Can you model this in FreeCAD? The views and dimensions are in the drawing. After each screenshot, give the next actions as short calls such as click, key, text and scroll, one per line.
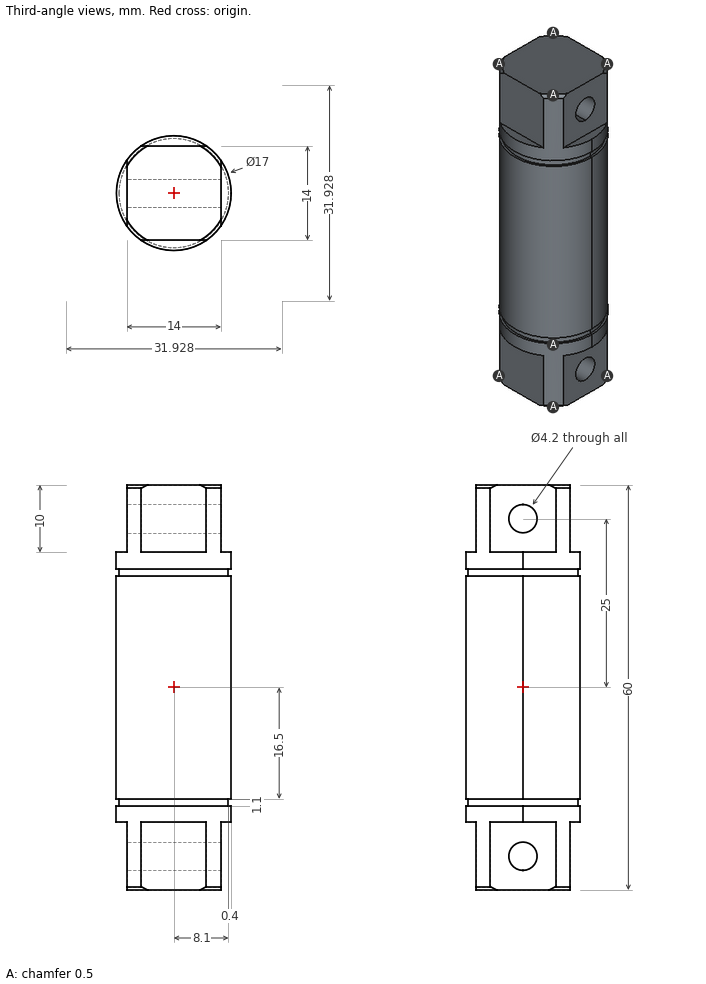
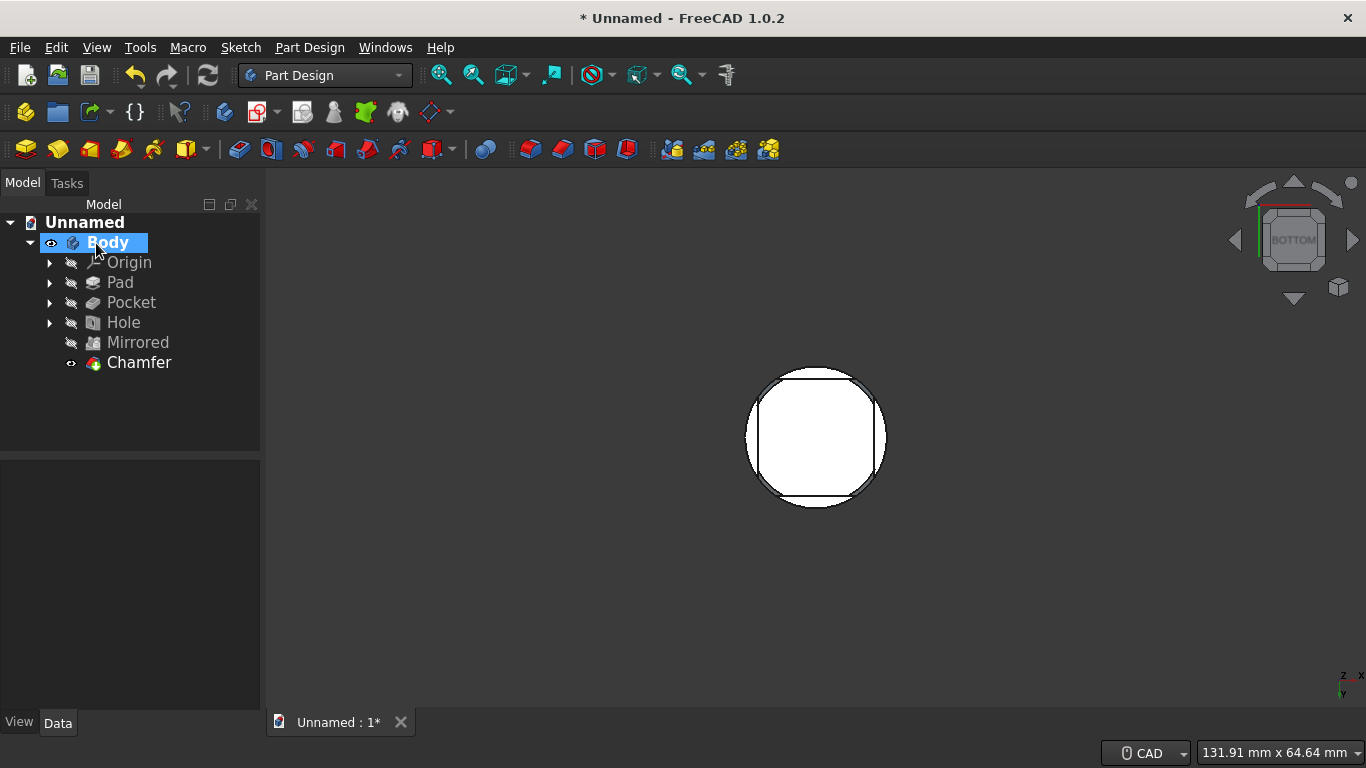
click(442, 76)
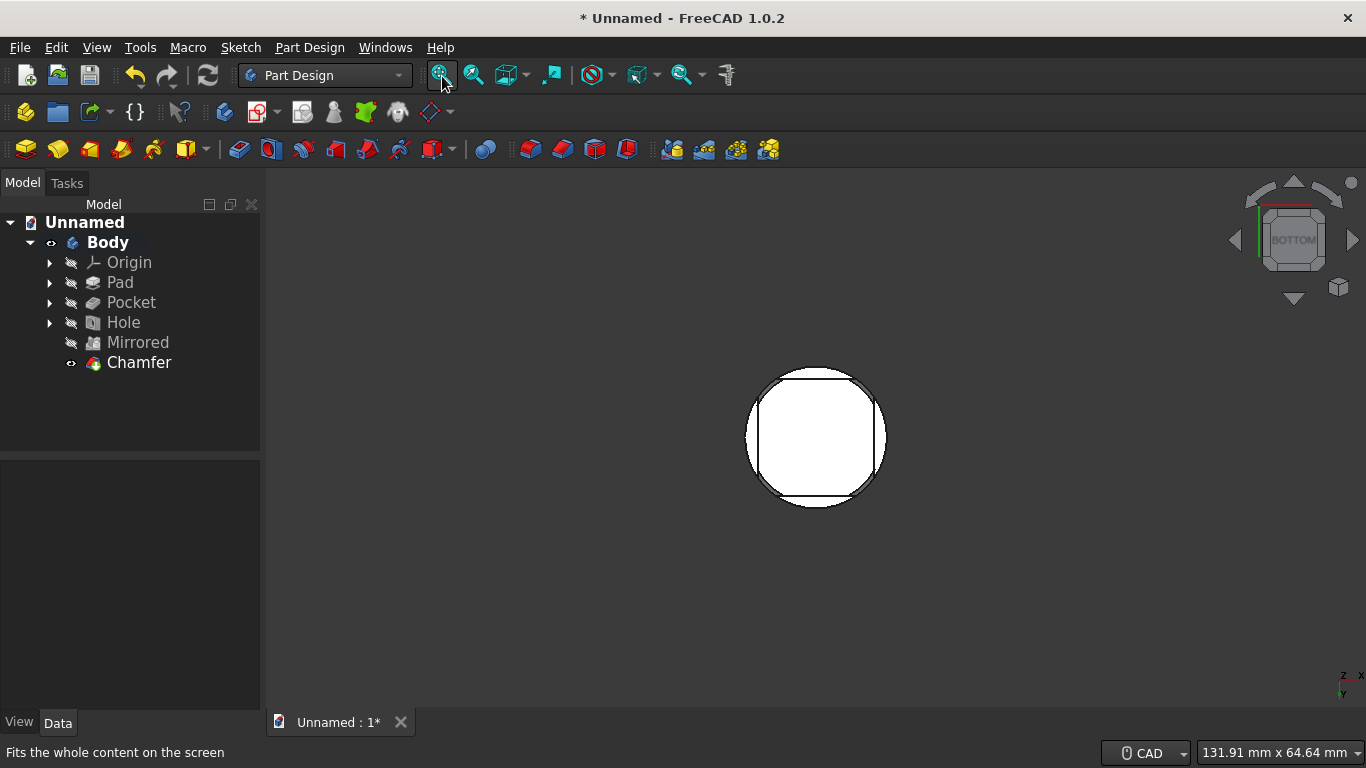
click(258, 112)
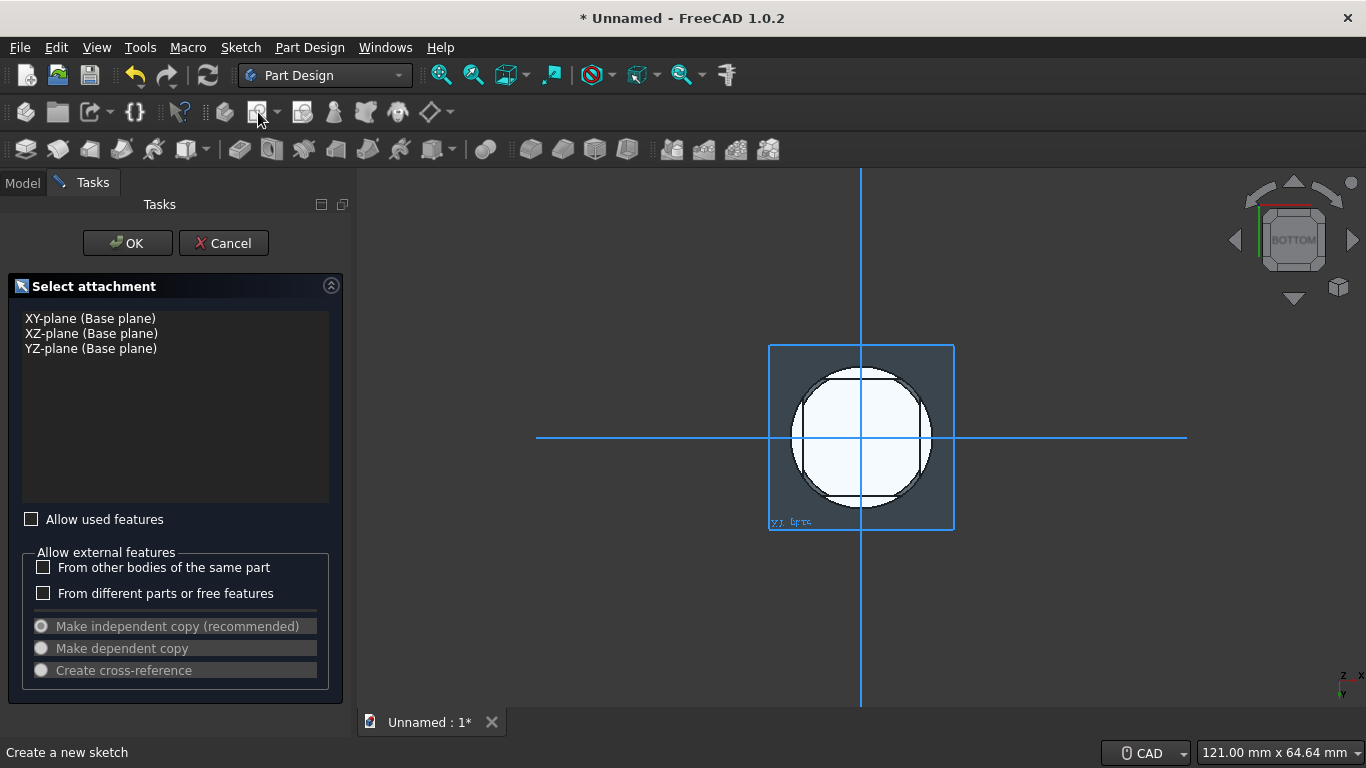
click(82, 334)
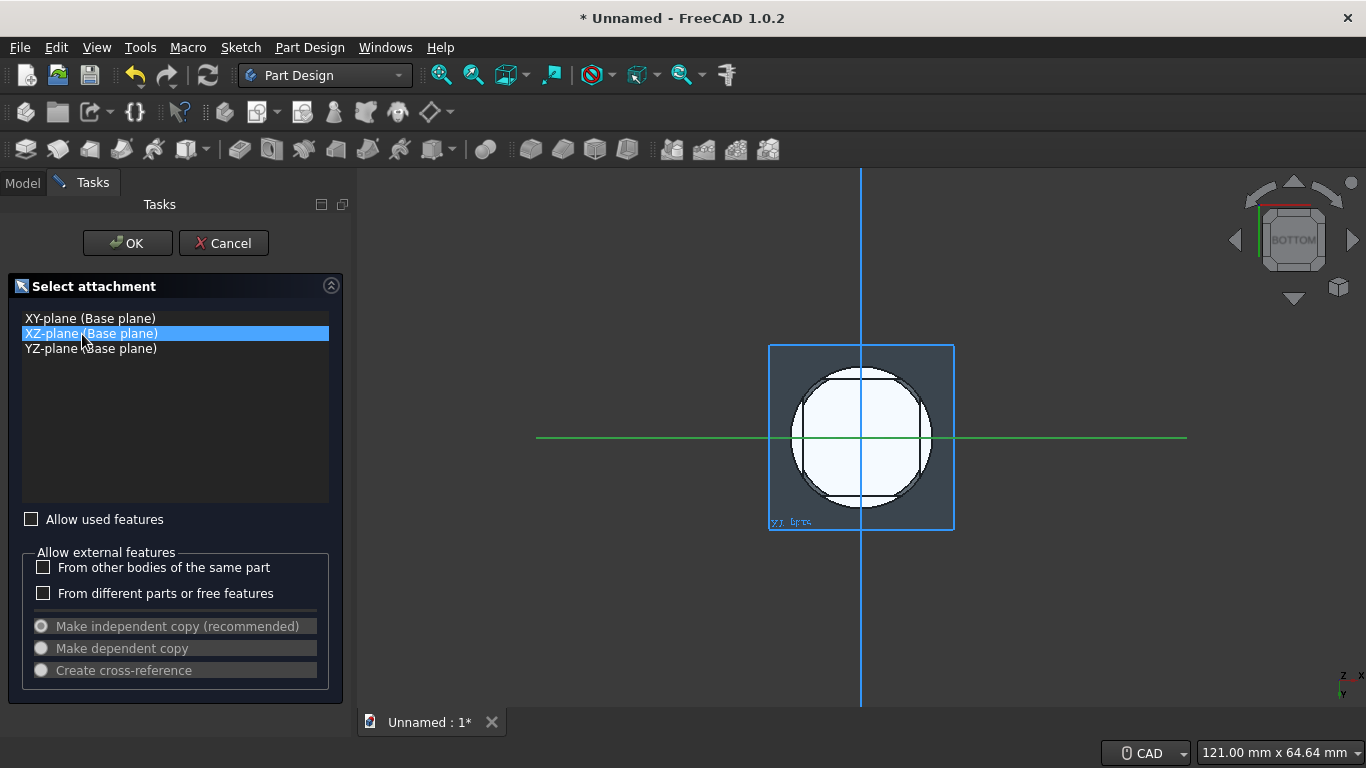
click(128, 243)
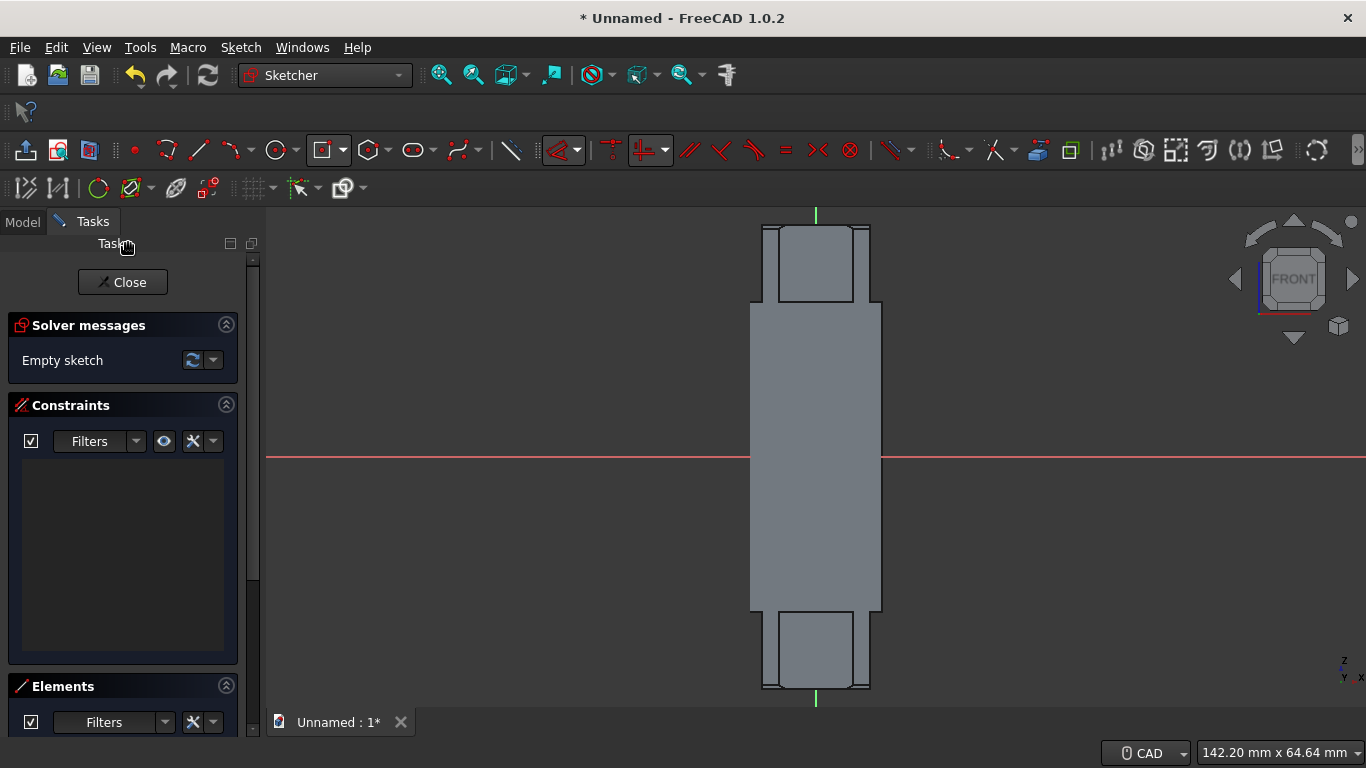
key(q)
key(s)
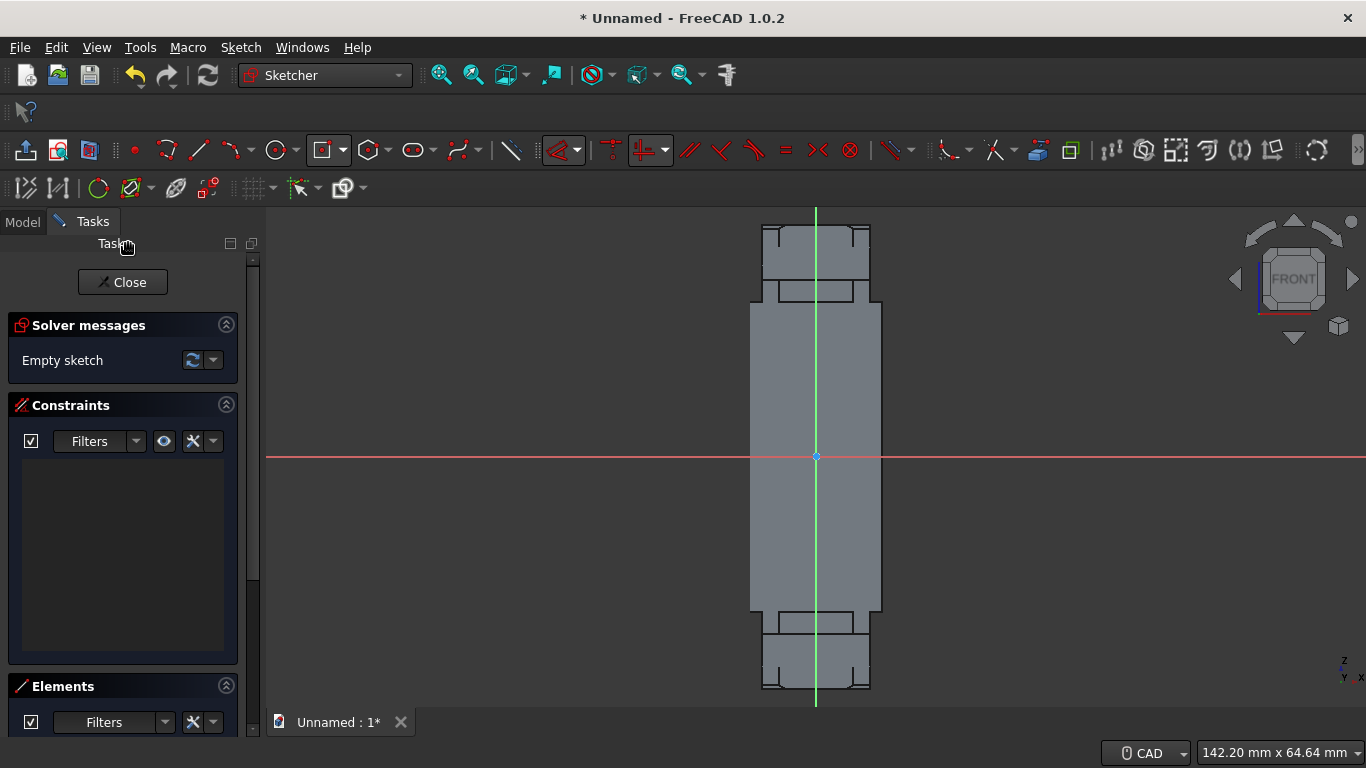
scroll(887, 596, up, 15)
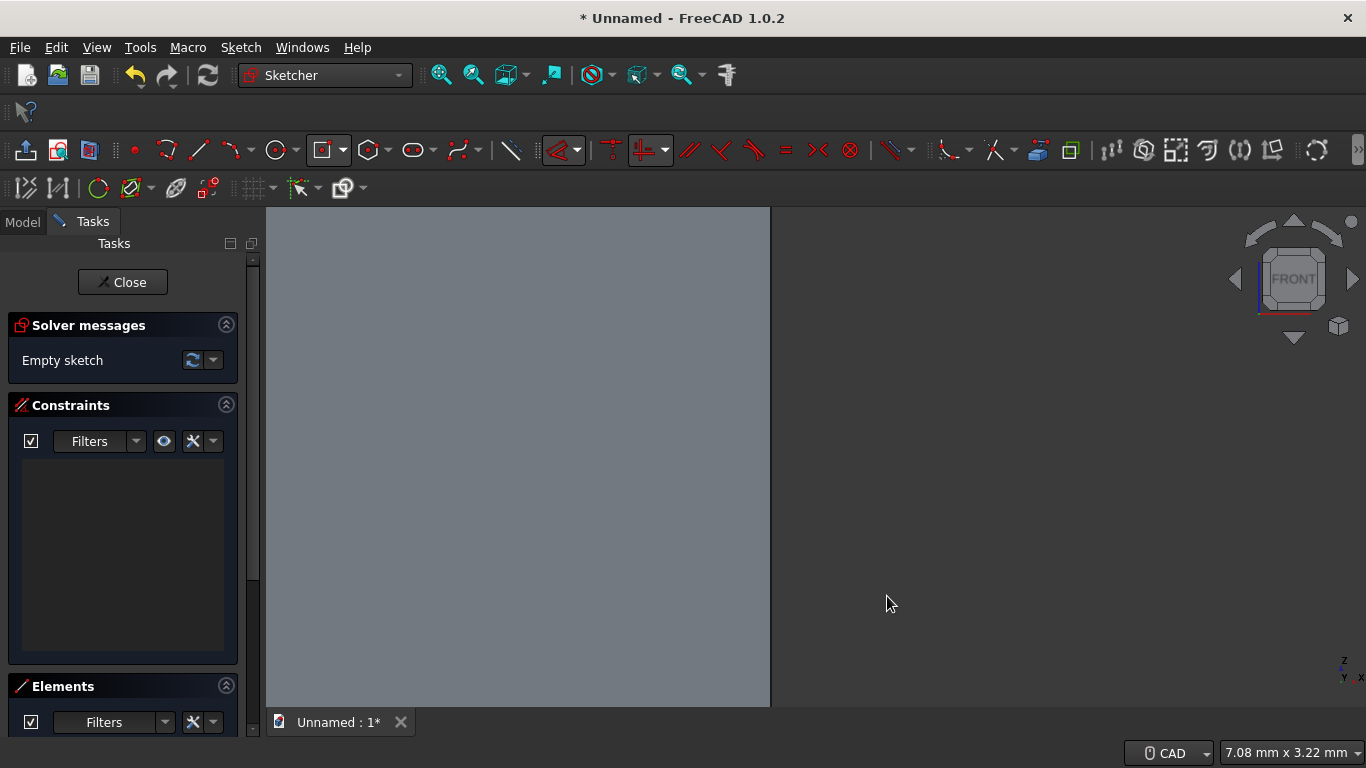
scroll(730, 416, up, 3)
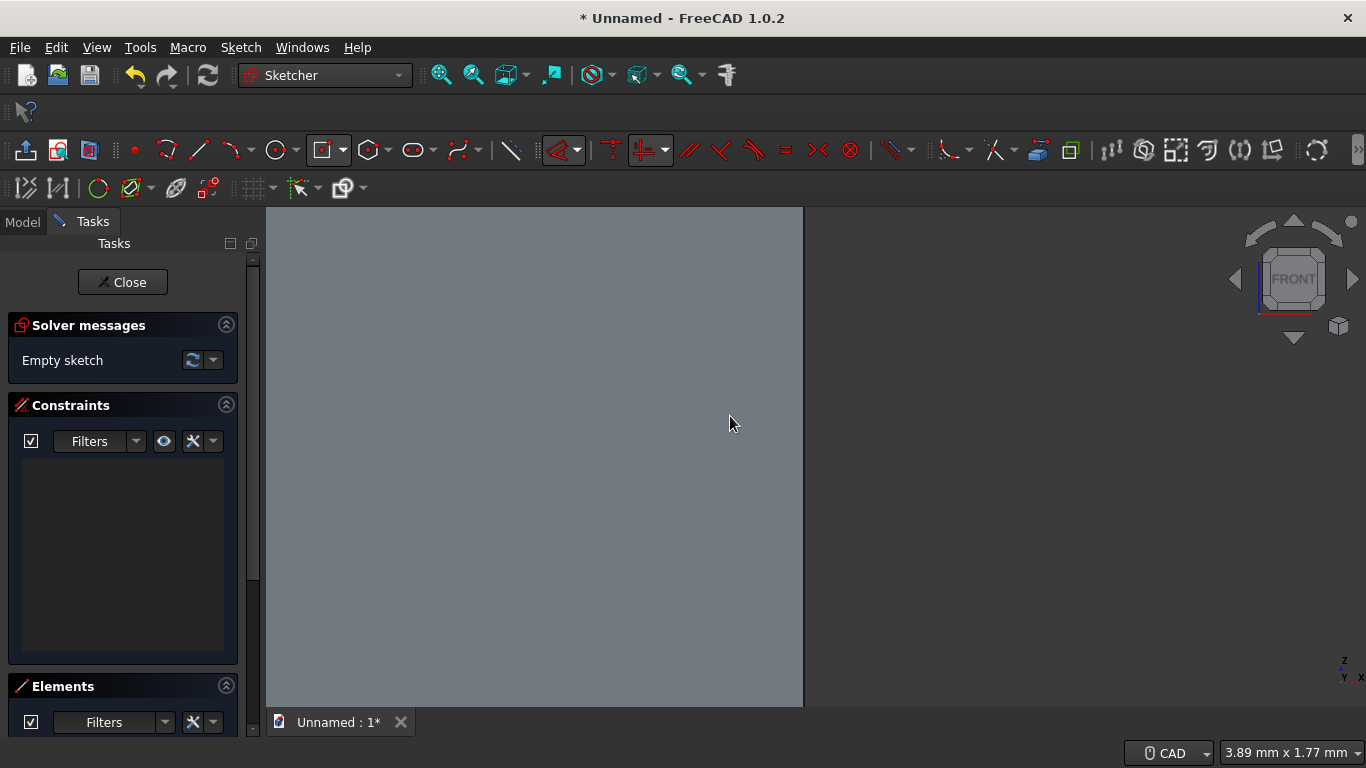
key(g)
key(r)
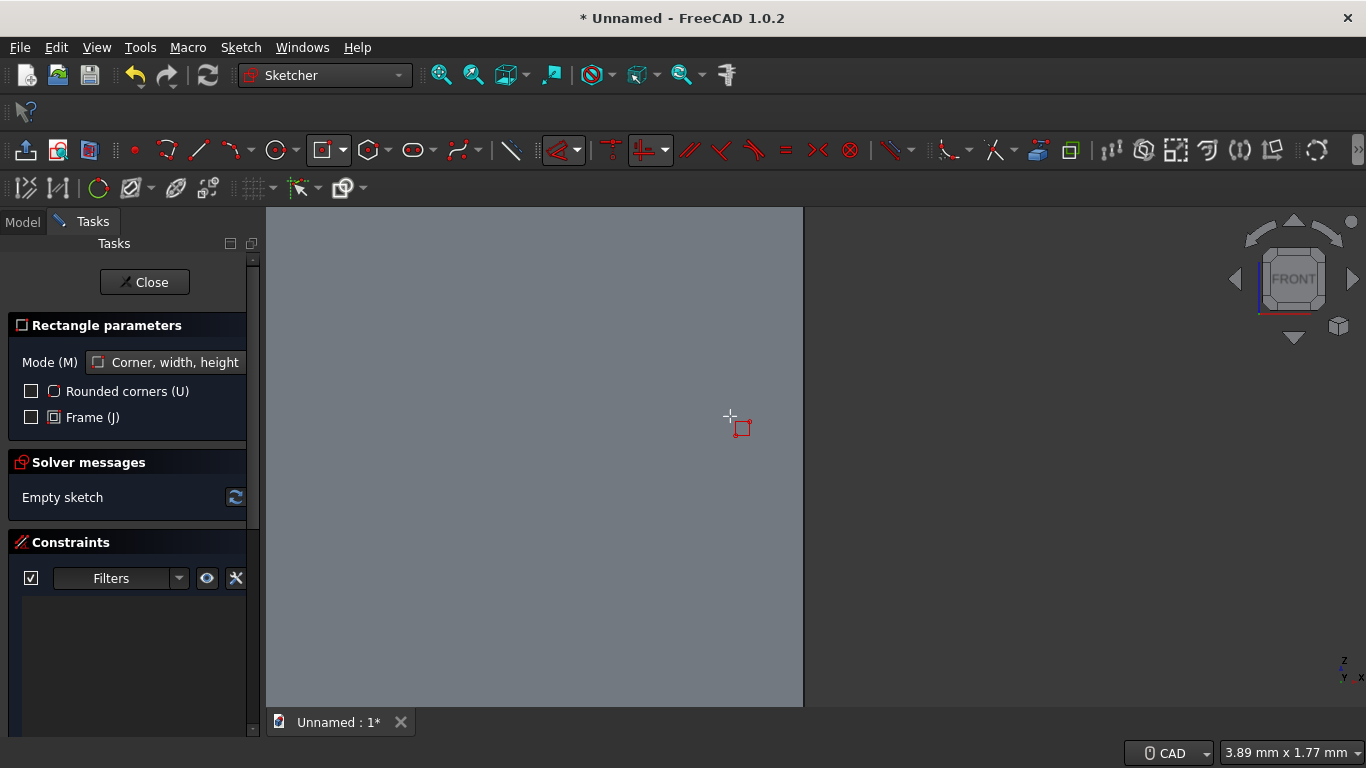
click(691, 301)
move(804, 612)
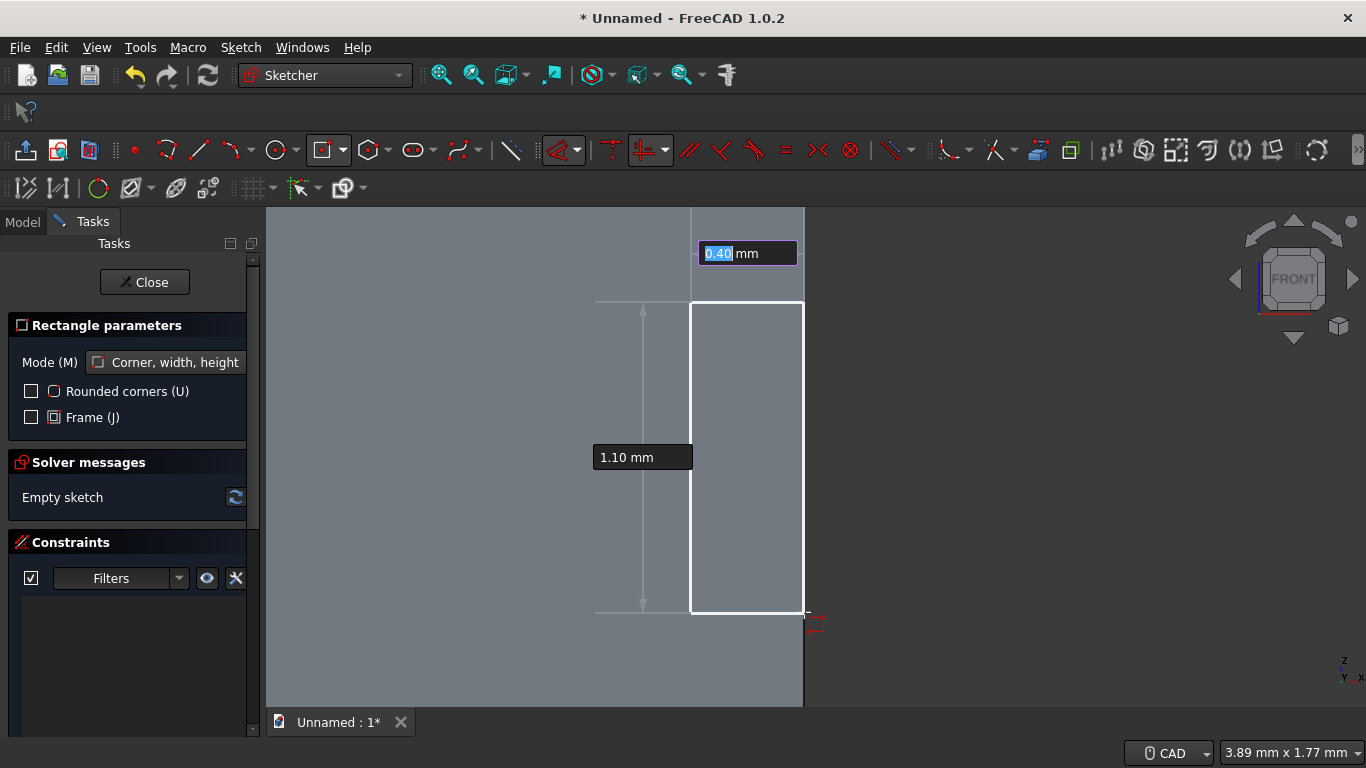
text(0.4)
key(Tab)
text(1.1)
key(Return)
key(Escape)